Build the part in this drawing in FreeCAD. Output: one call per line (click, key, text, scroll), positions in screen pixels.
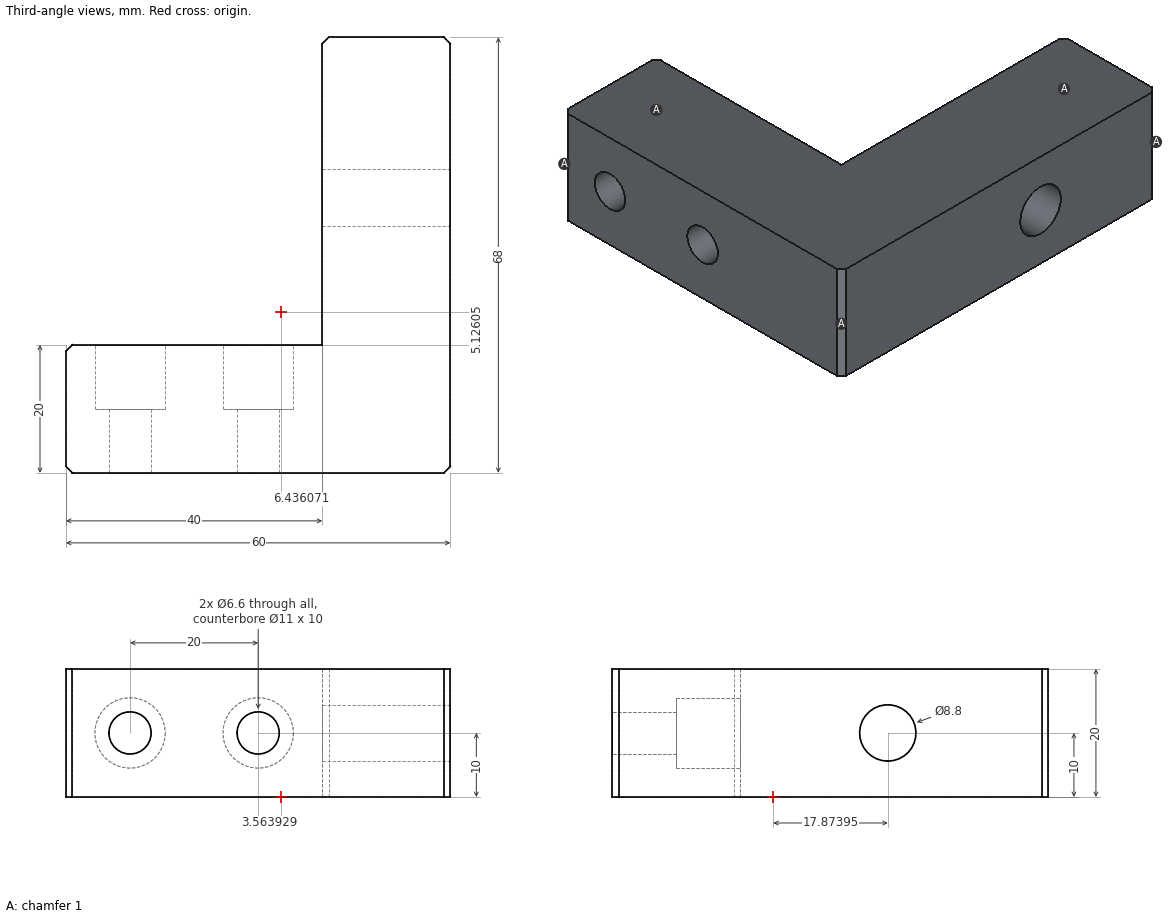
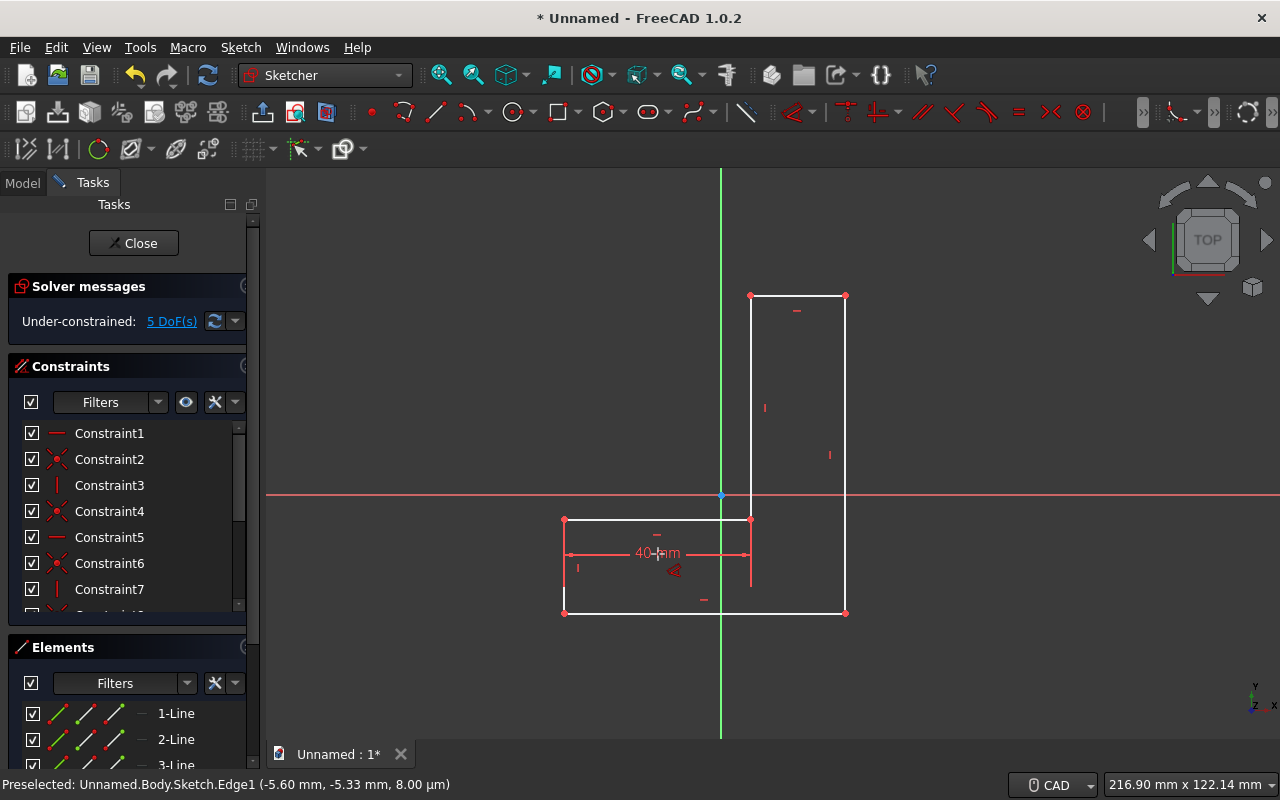
click(564, 548)
click(530, 567)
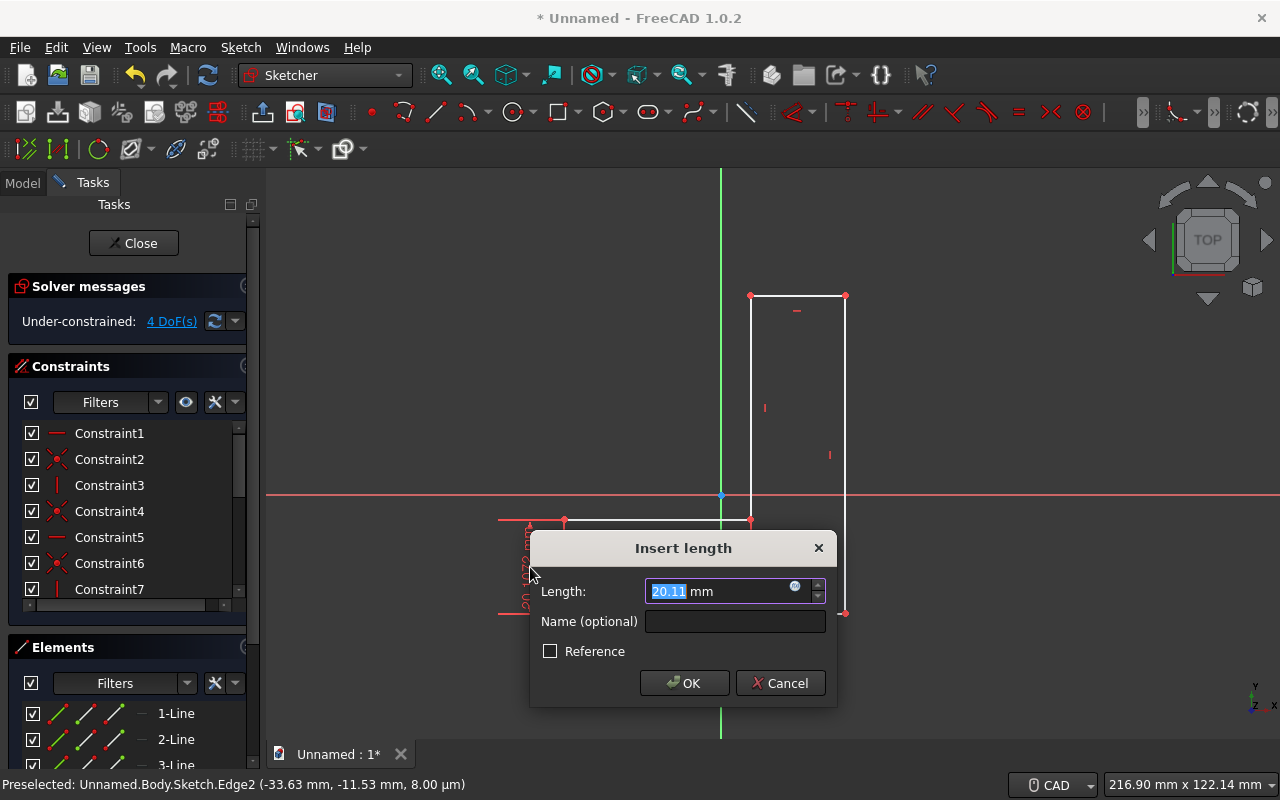
text(20)
key(Return)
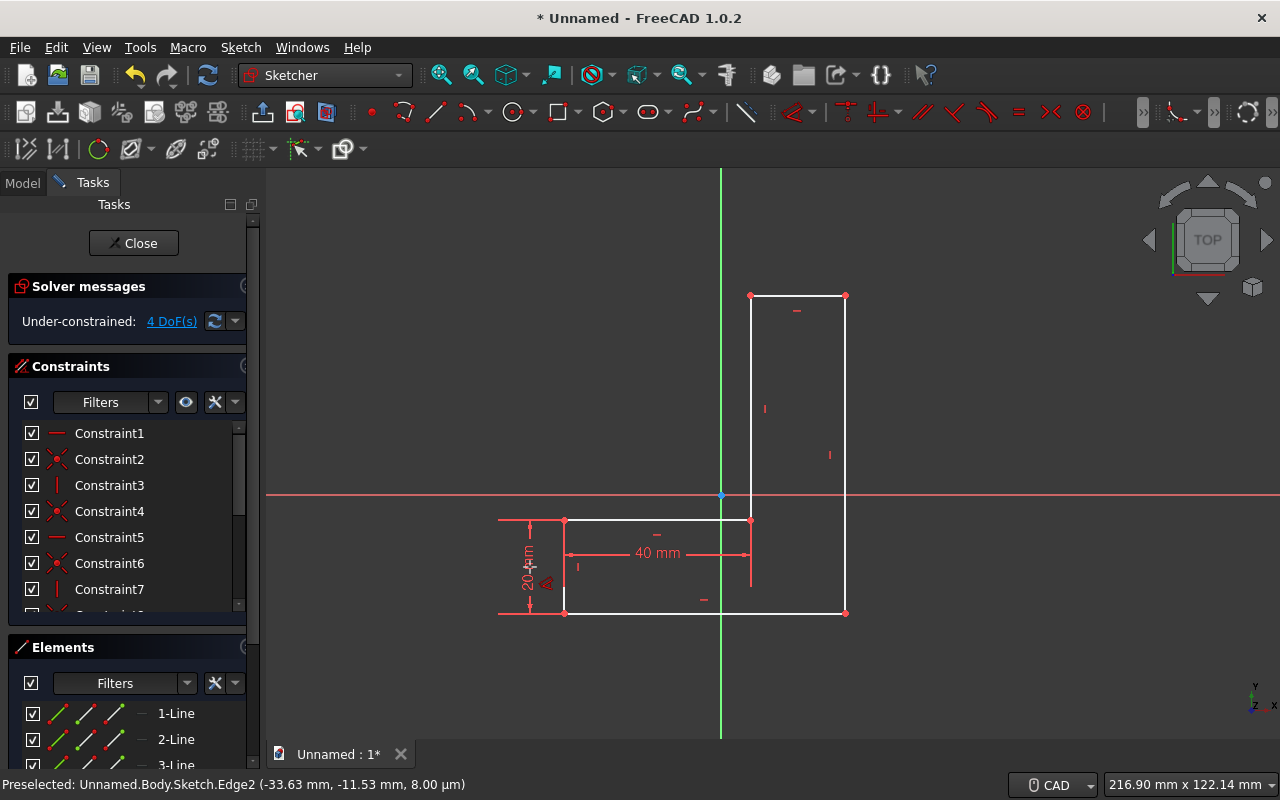
click(648, 614)
click(704, 648)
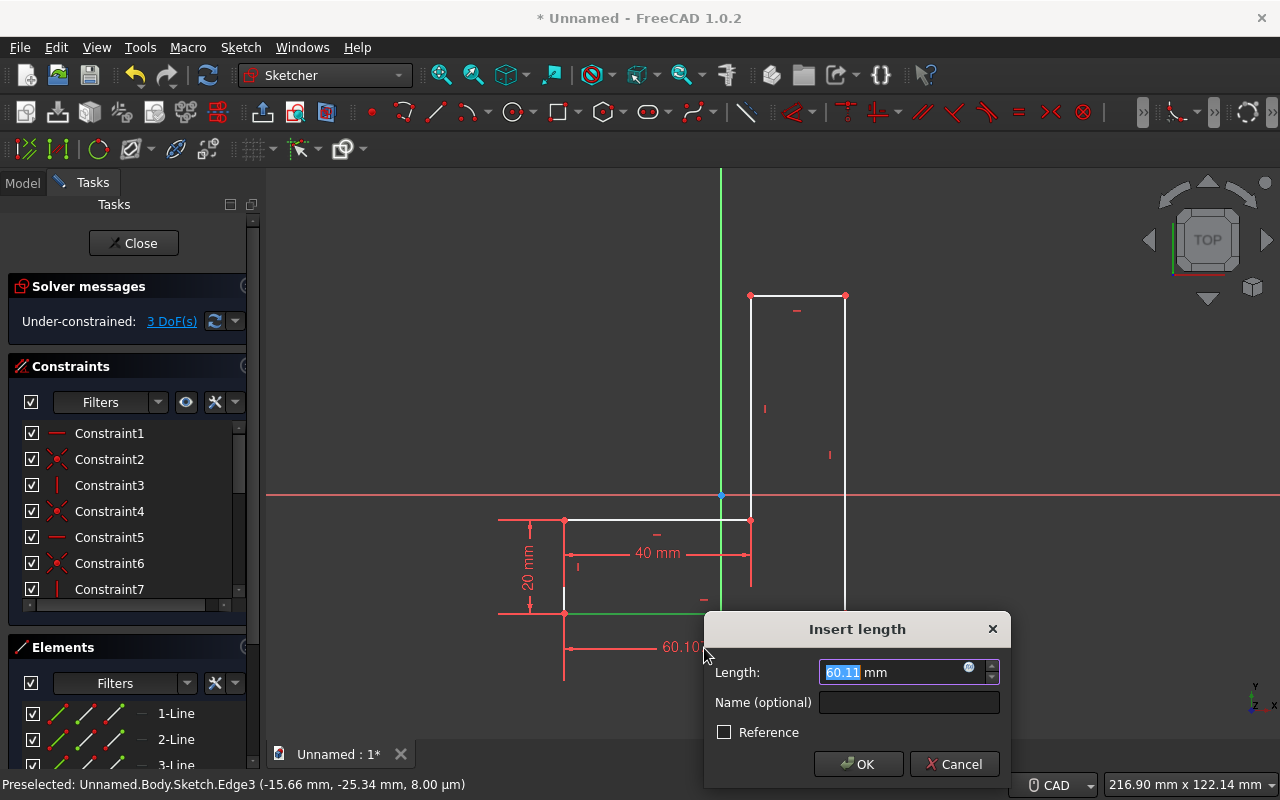
text(60)
key(Return)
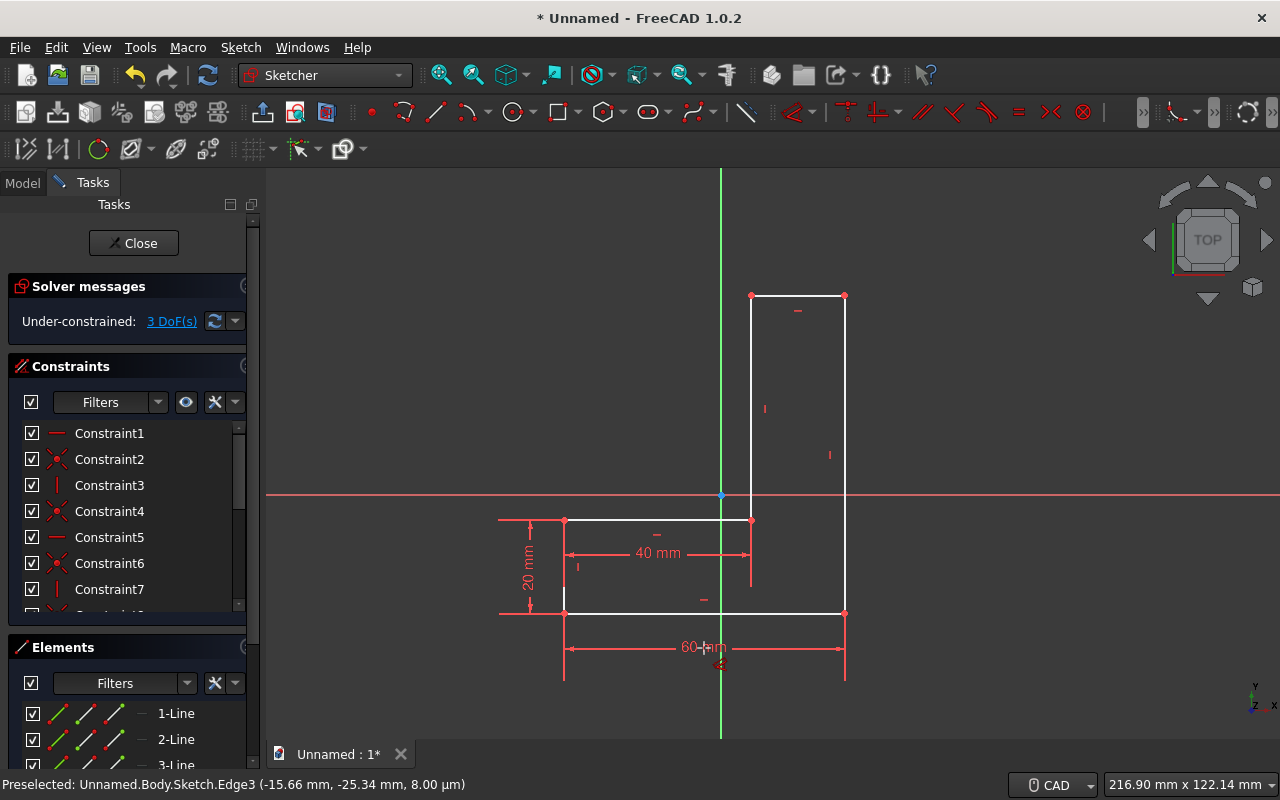
click(845, 518)
click(879, 455)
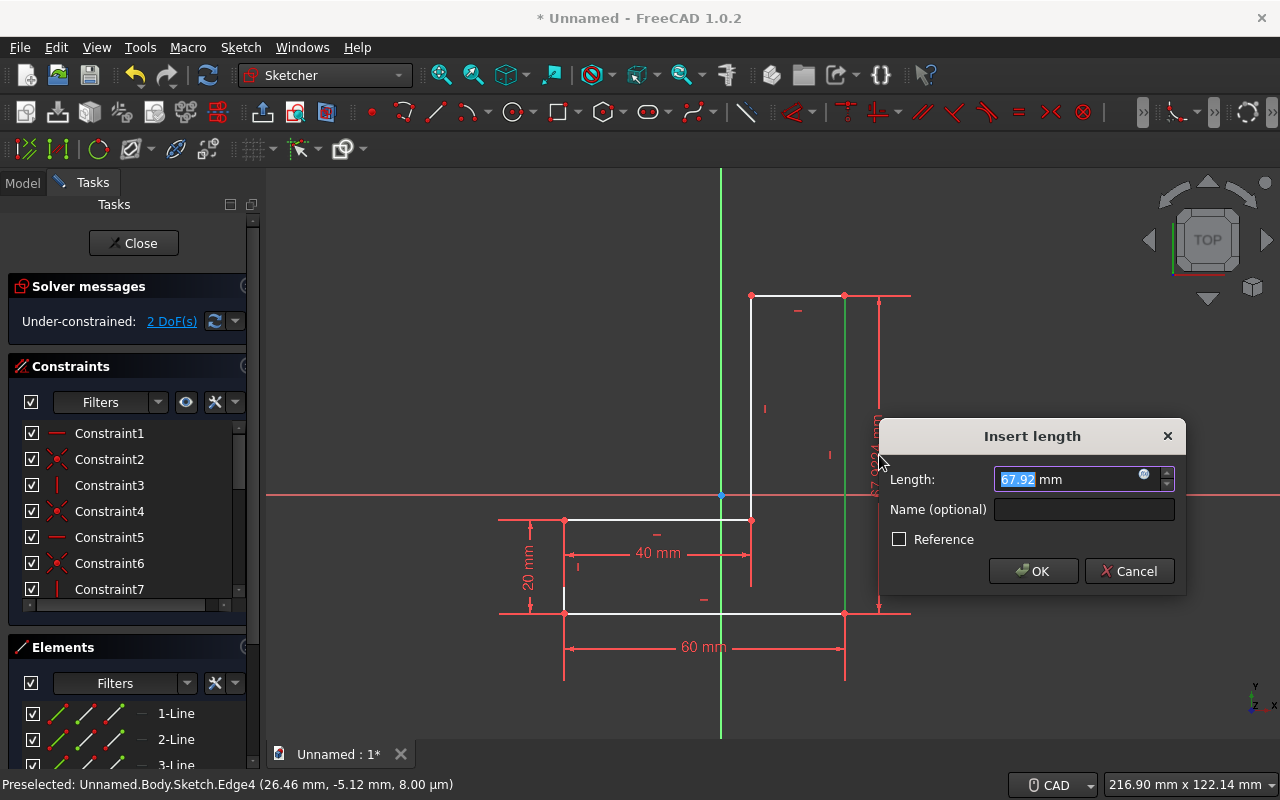
text(68)
key(Return)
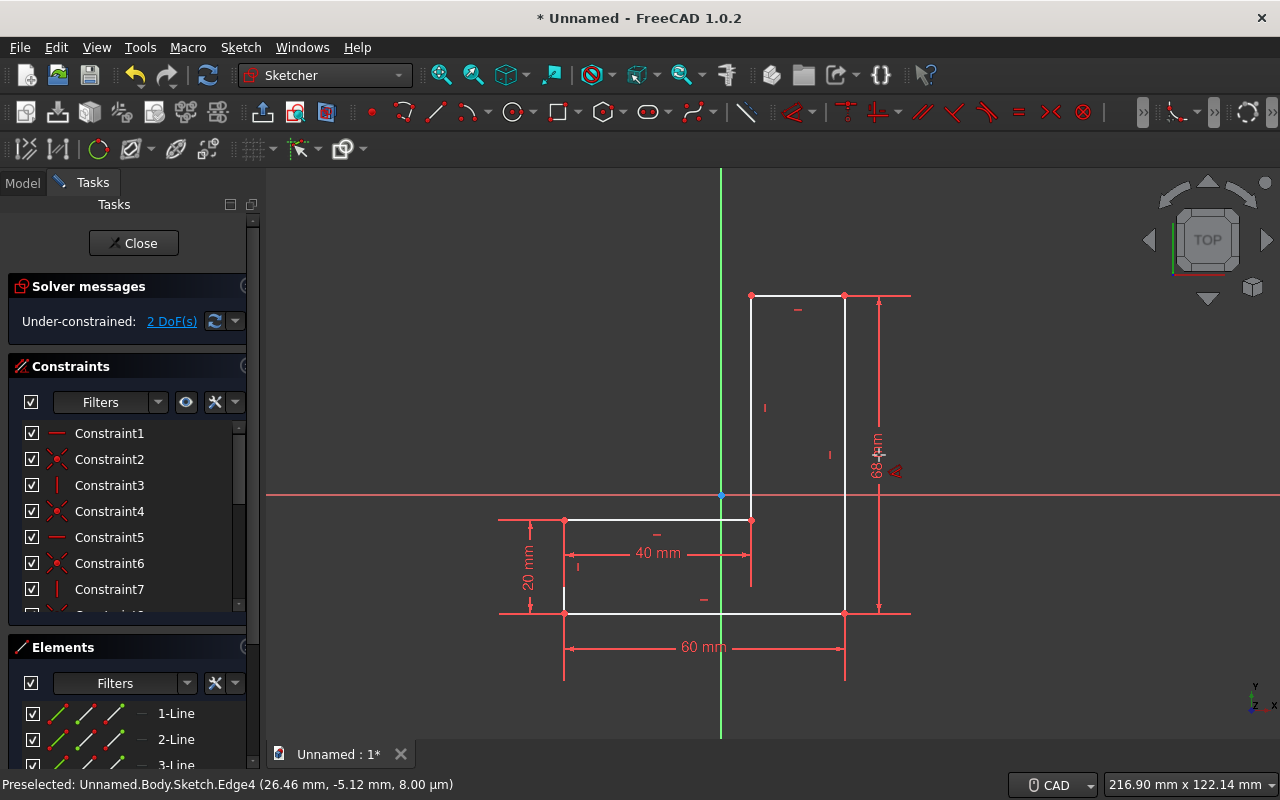
scroll(751, 520, up, 3)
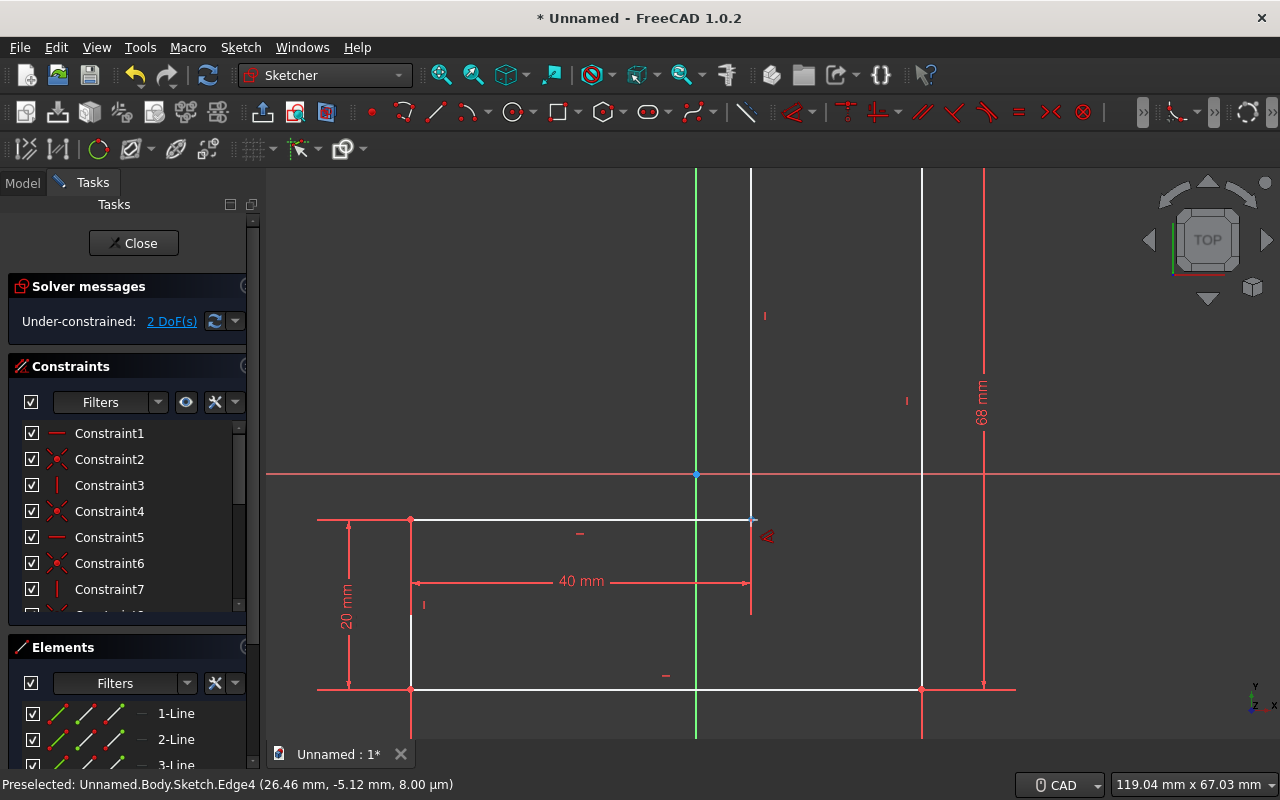
click(751, 520)
click(785, 497)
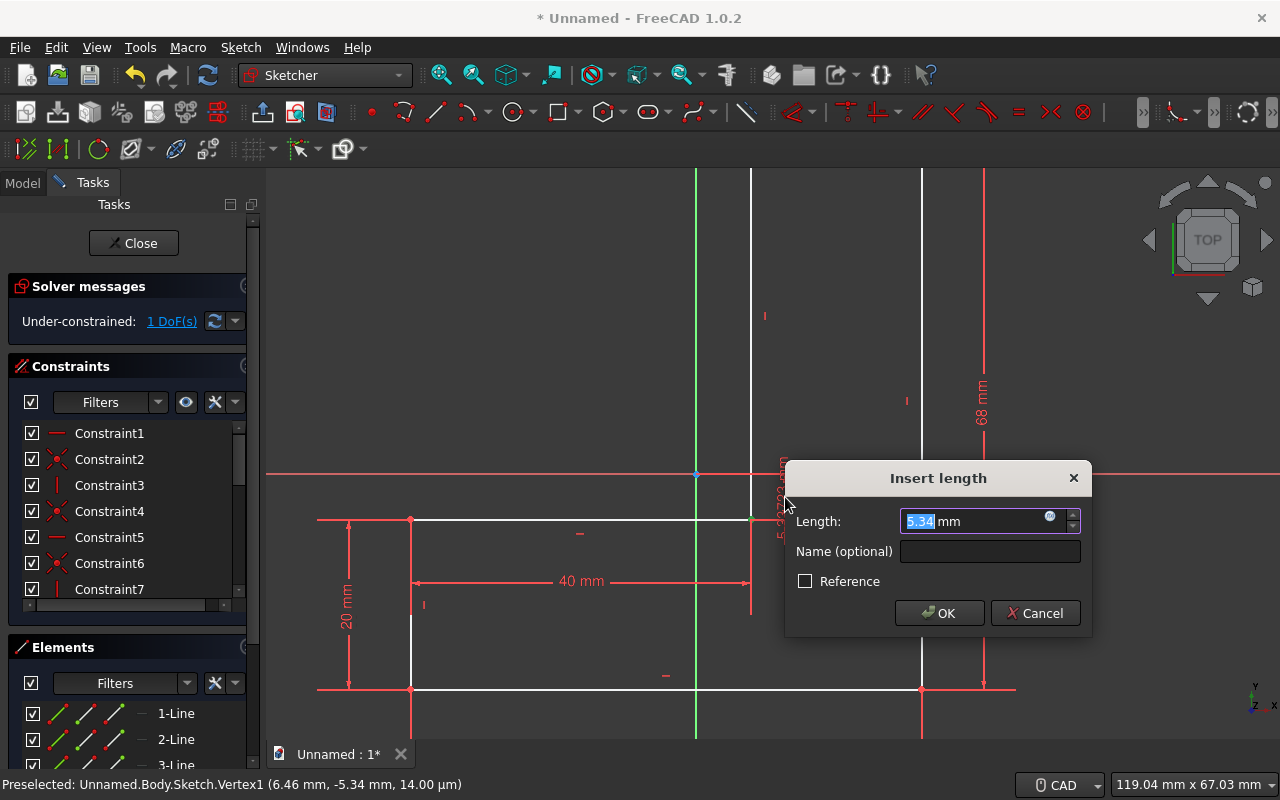
text(5.12605)
key(Return)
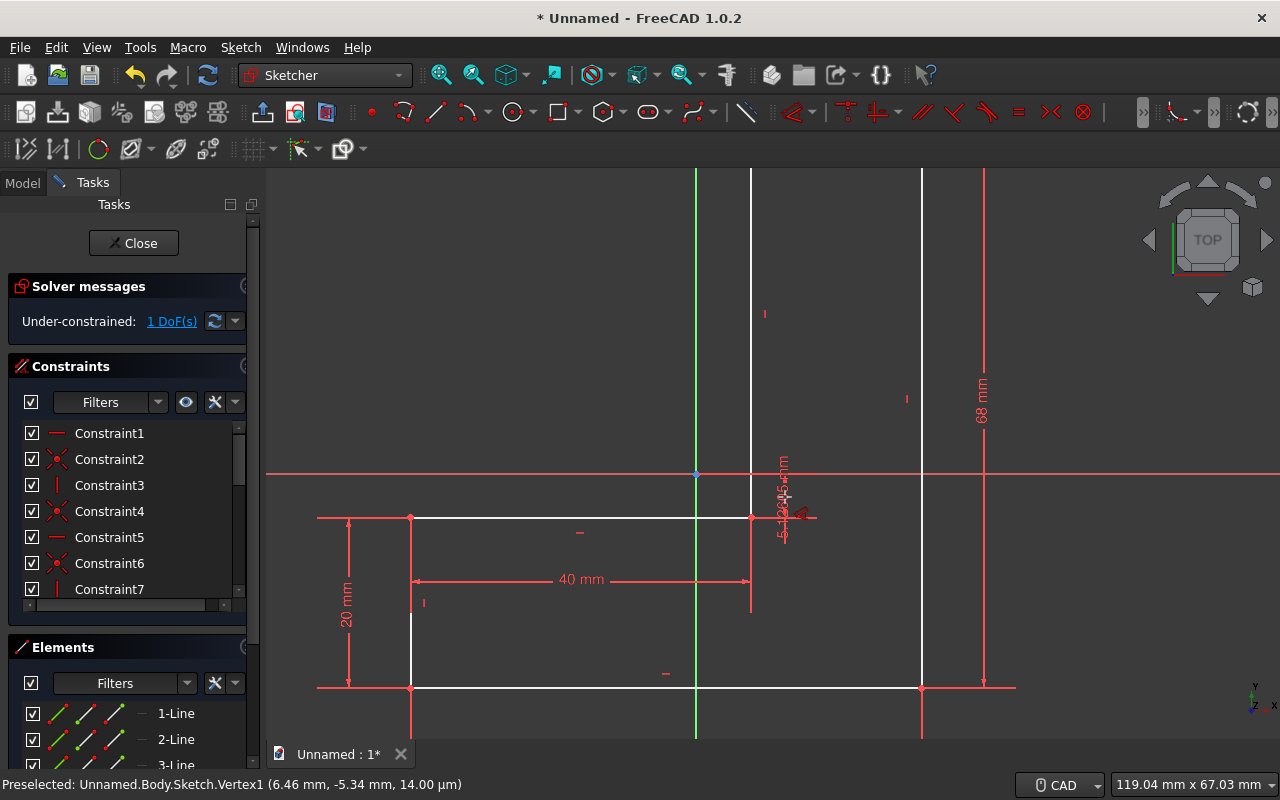
click(751, 518)
click(724, 552)